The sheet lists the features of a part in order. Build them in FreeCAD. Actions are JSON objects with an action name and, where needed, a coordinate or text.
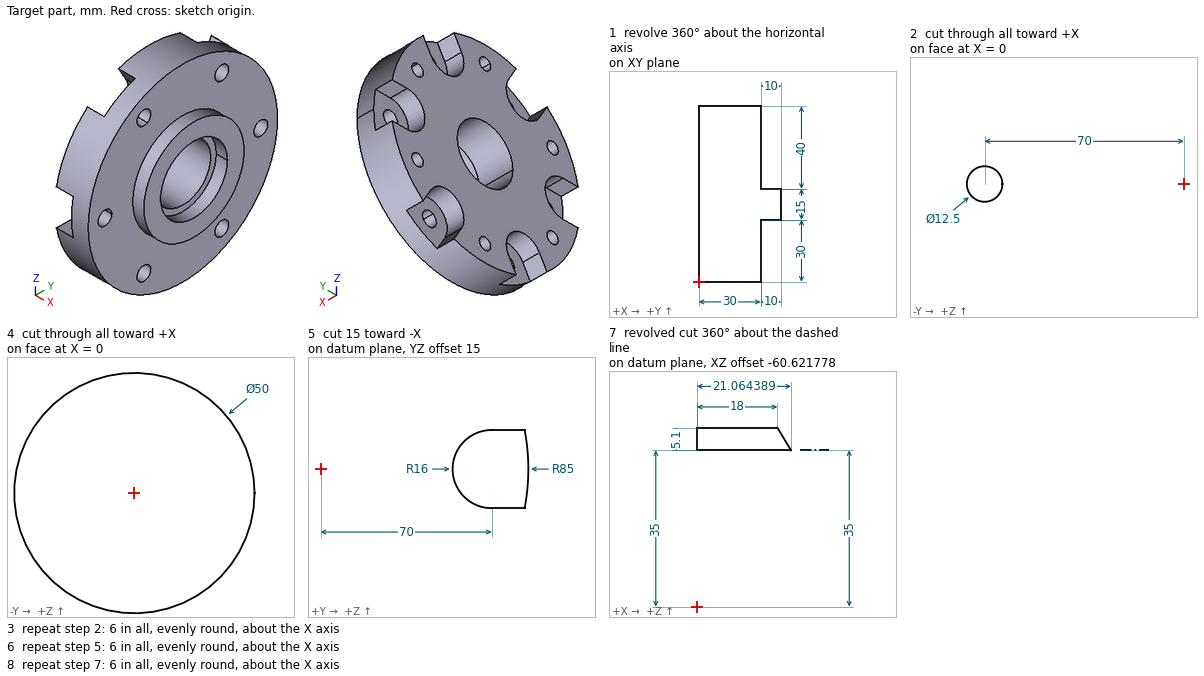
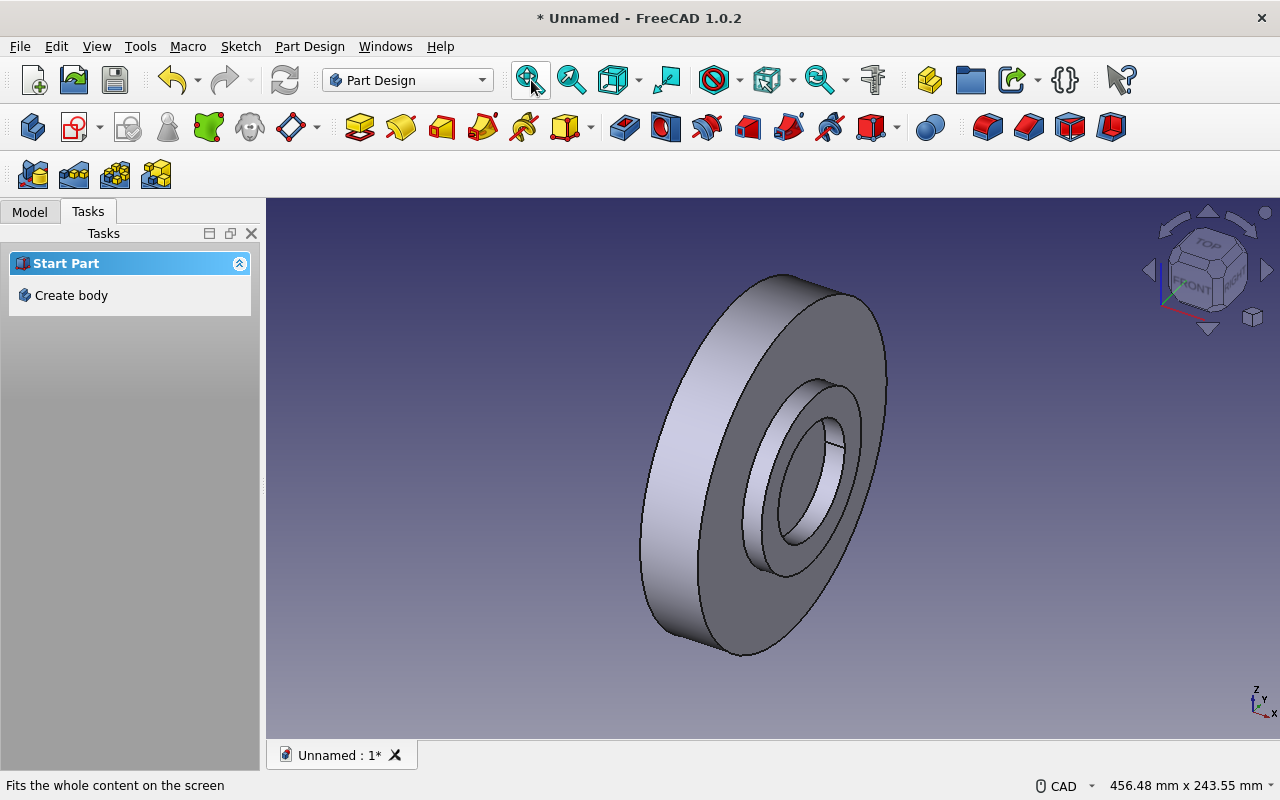
{"action": "key", "text": "6"}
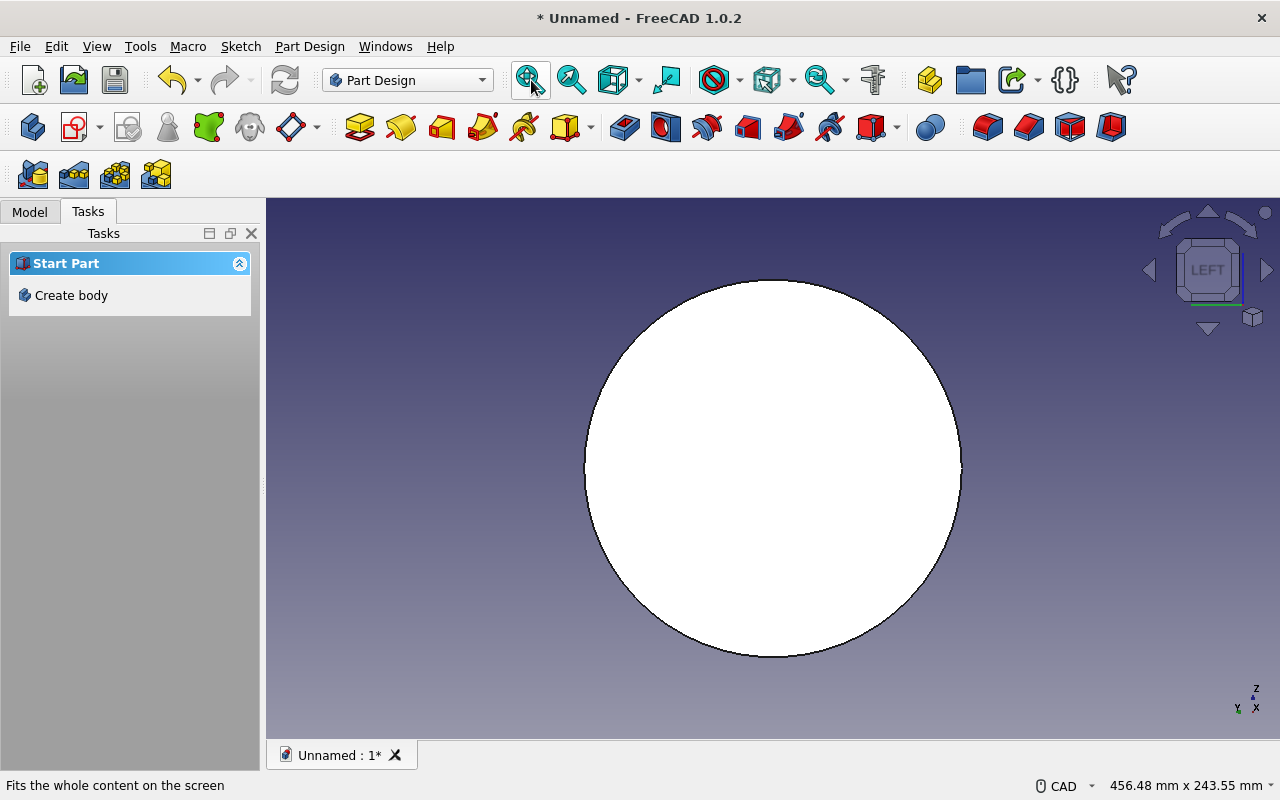
{"action": "left_click", "coordinate": [773, 467]}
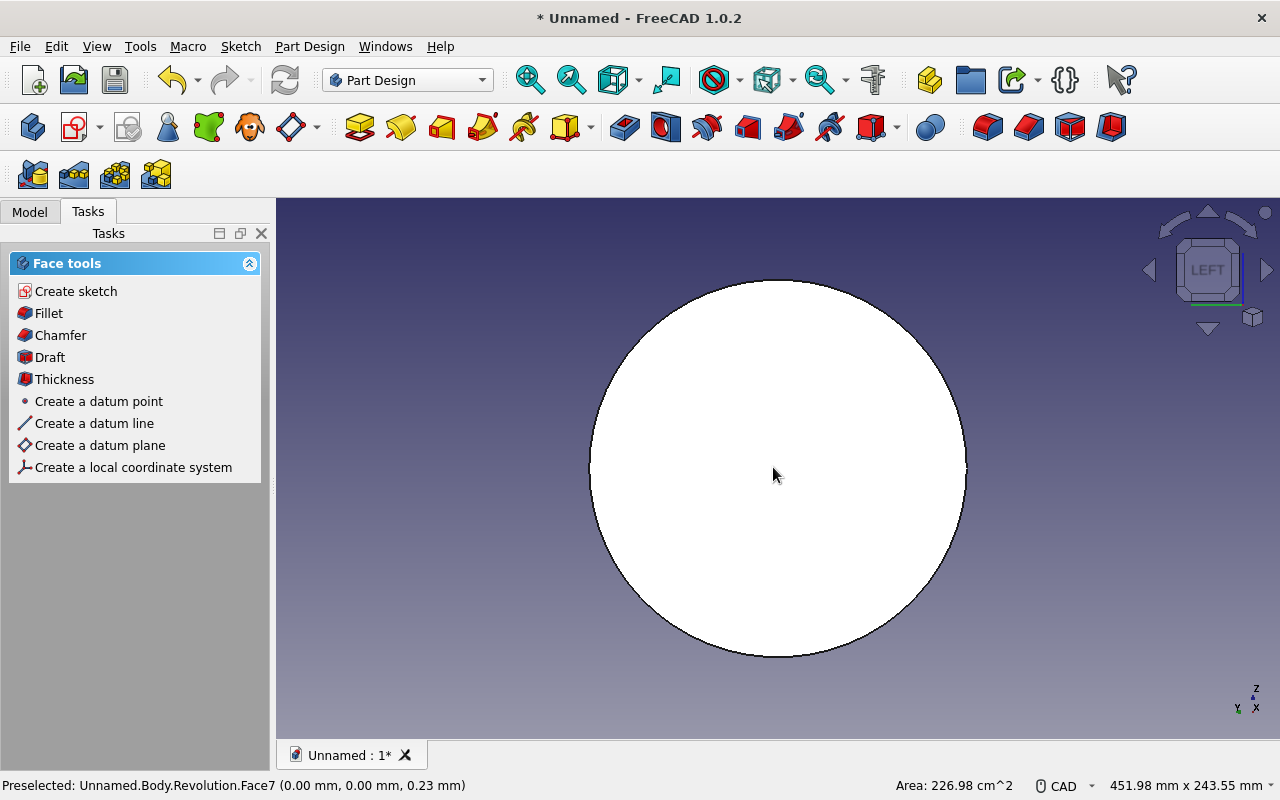
{"action": "left_click", "coordinate": [74, 128]}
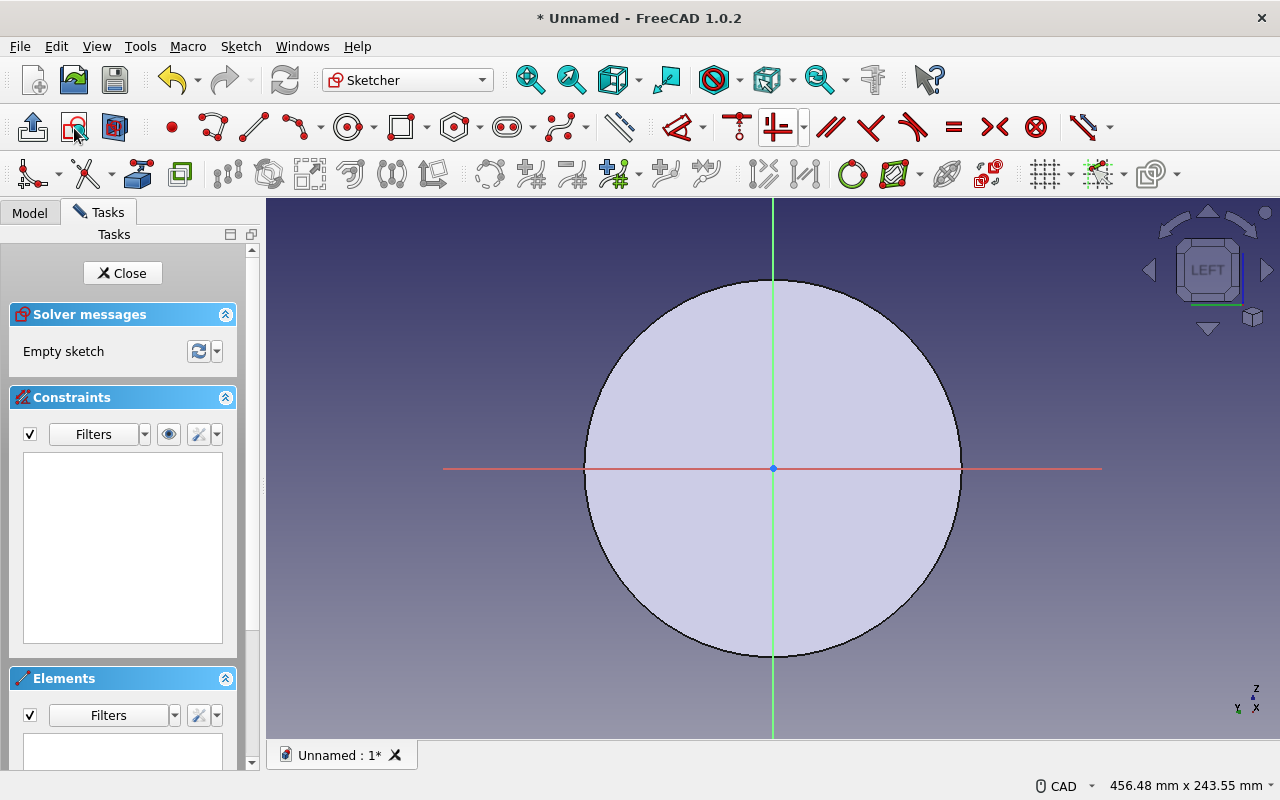
{"action": "scroll", "coordinate": [611, 468], "scroll_direction": "up", "scroll_amount": 13}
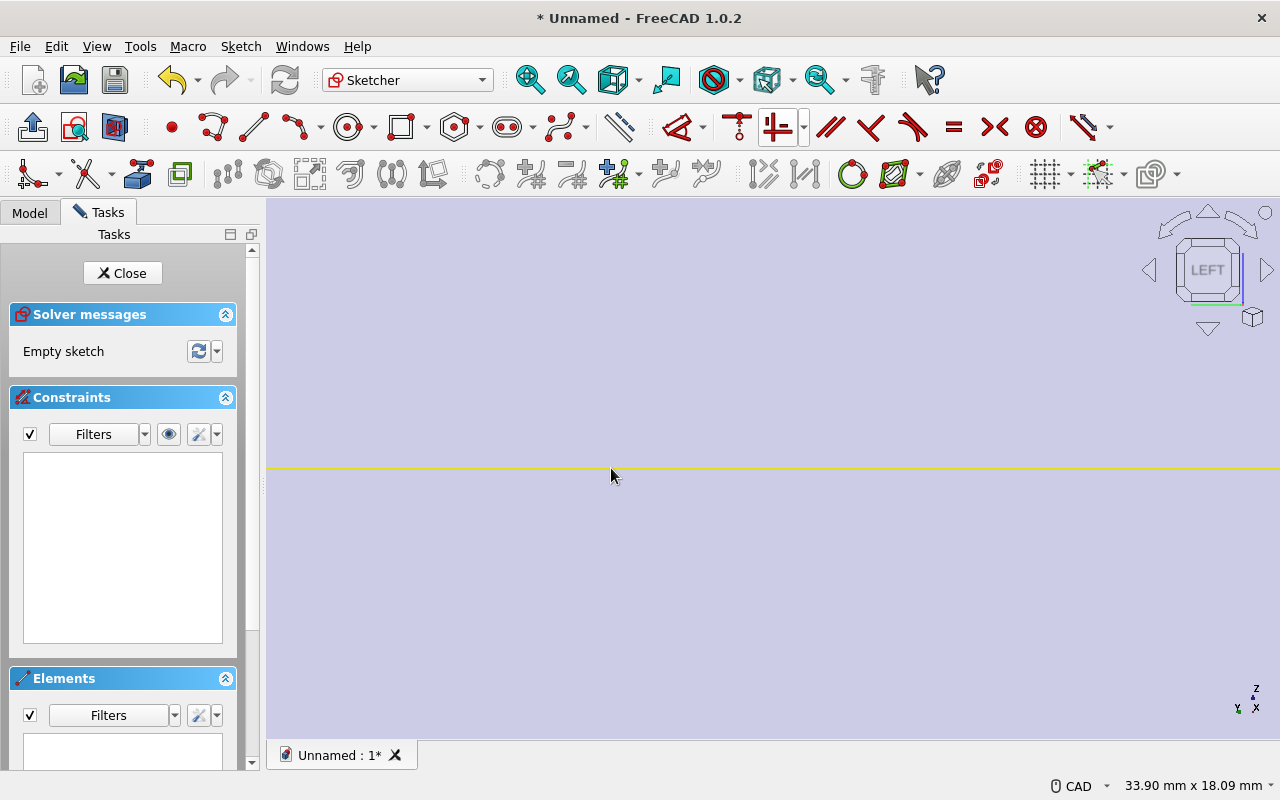
{"action": "left_click", "coordinate": [348, 128]}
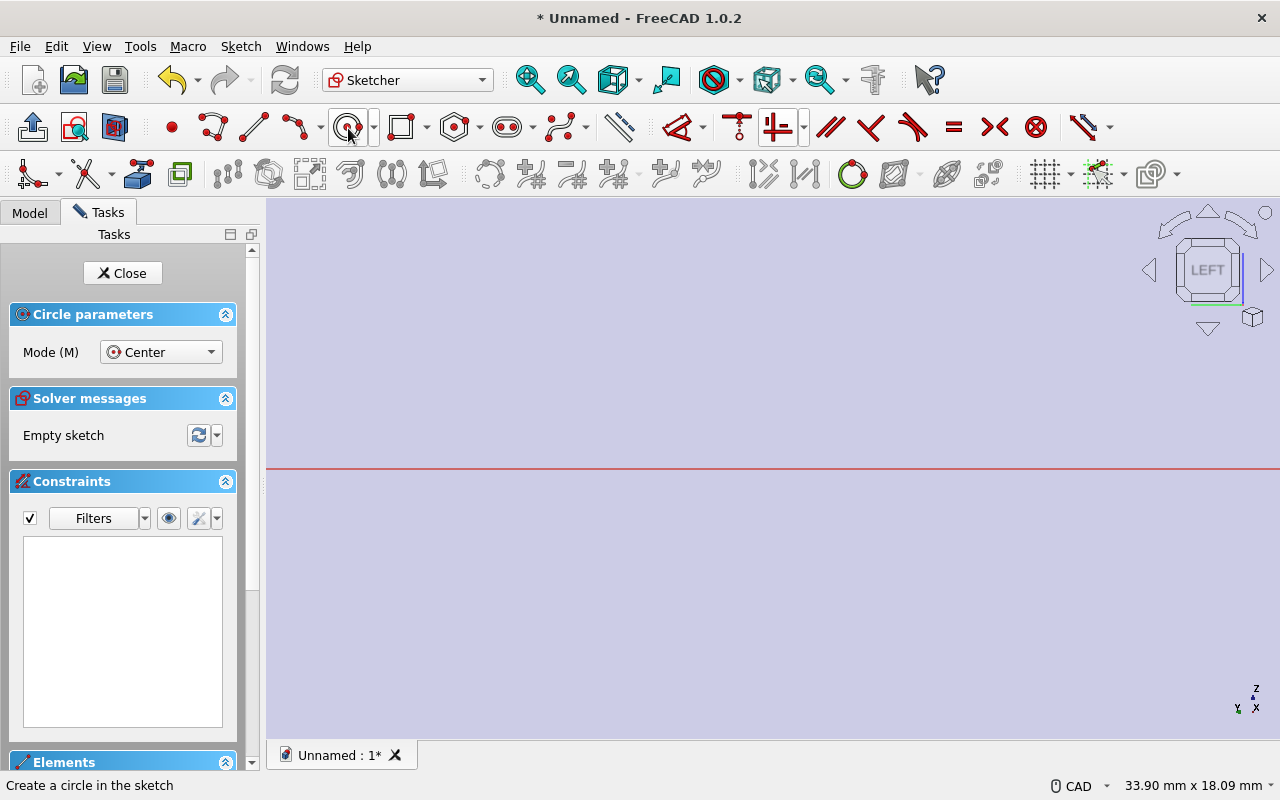
{"action": "left_click", "coordinate": [694, 468]}
{"action": "left_click", "coordinate": [827, 336]}
{"action": "key", "text": "Escape"}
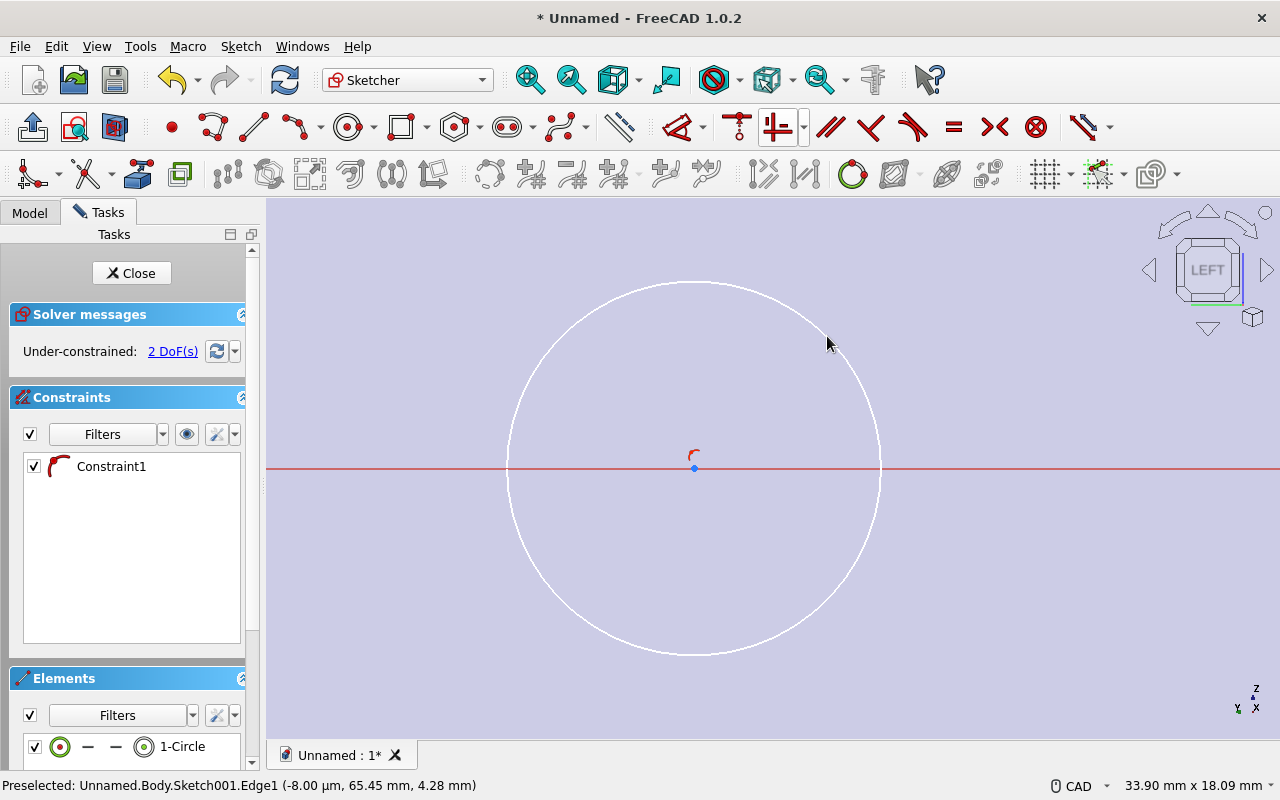
{"action": "left_click", "coordinate": [676, 128]}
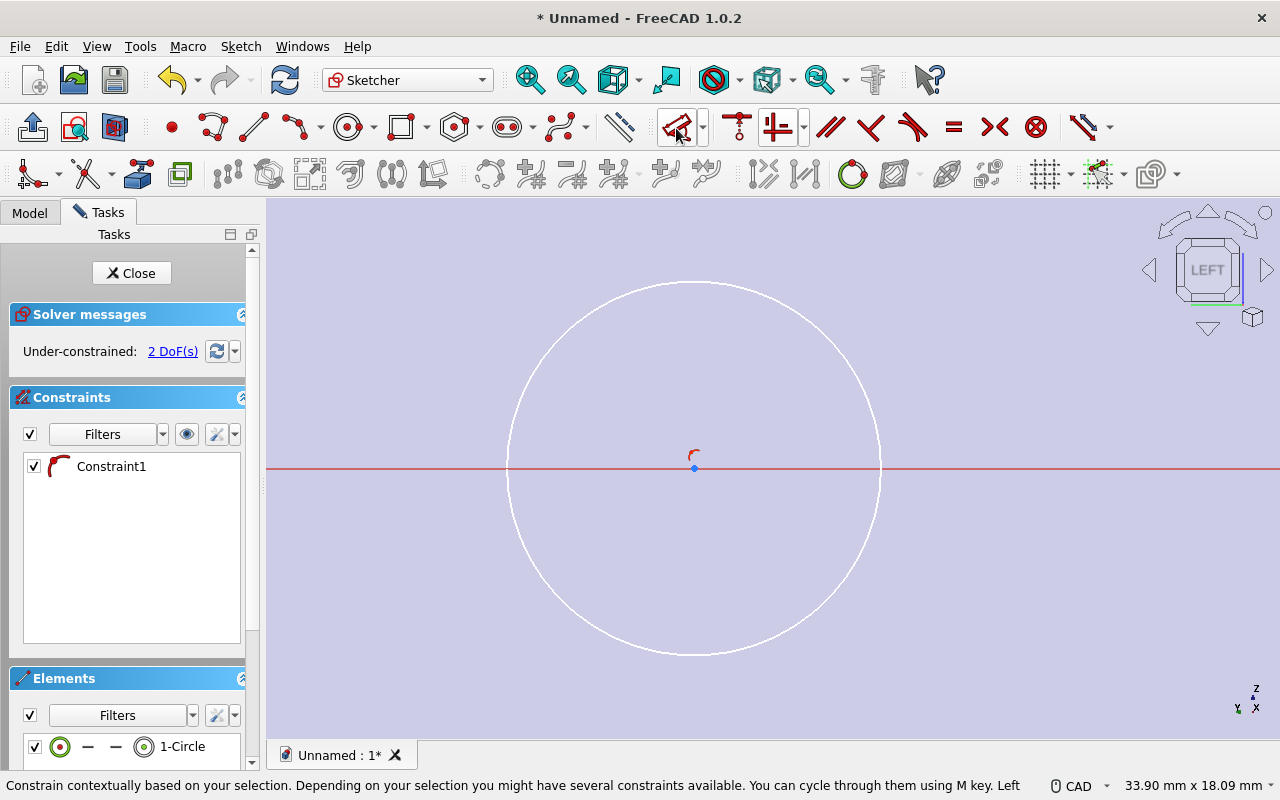
{"action": "left_click", "coordinate": [826, 336]}
{"action": "left_click", "coordinate": [849, 313]}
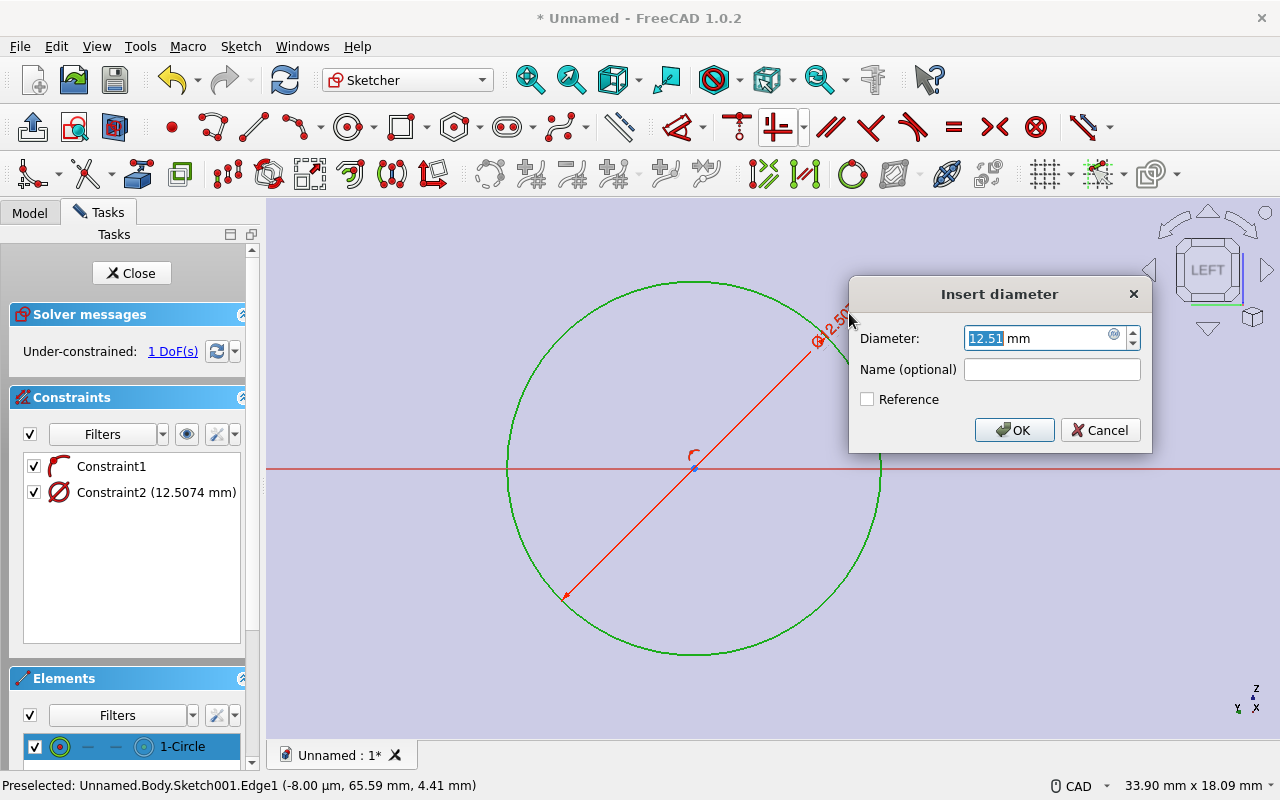
{"action": "type", "text": "12.5"}
{"action": "key", "text": "Return"}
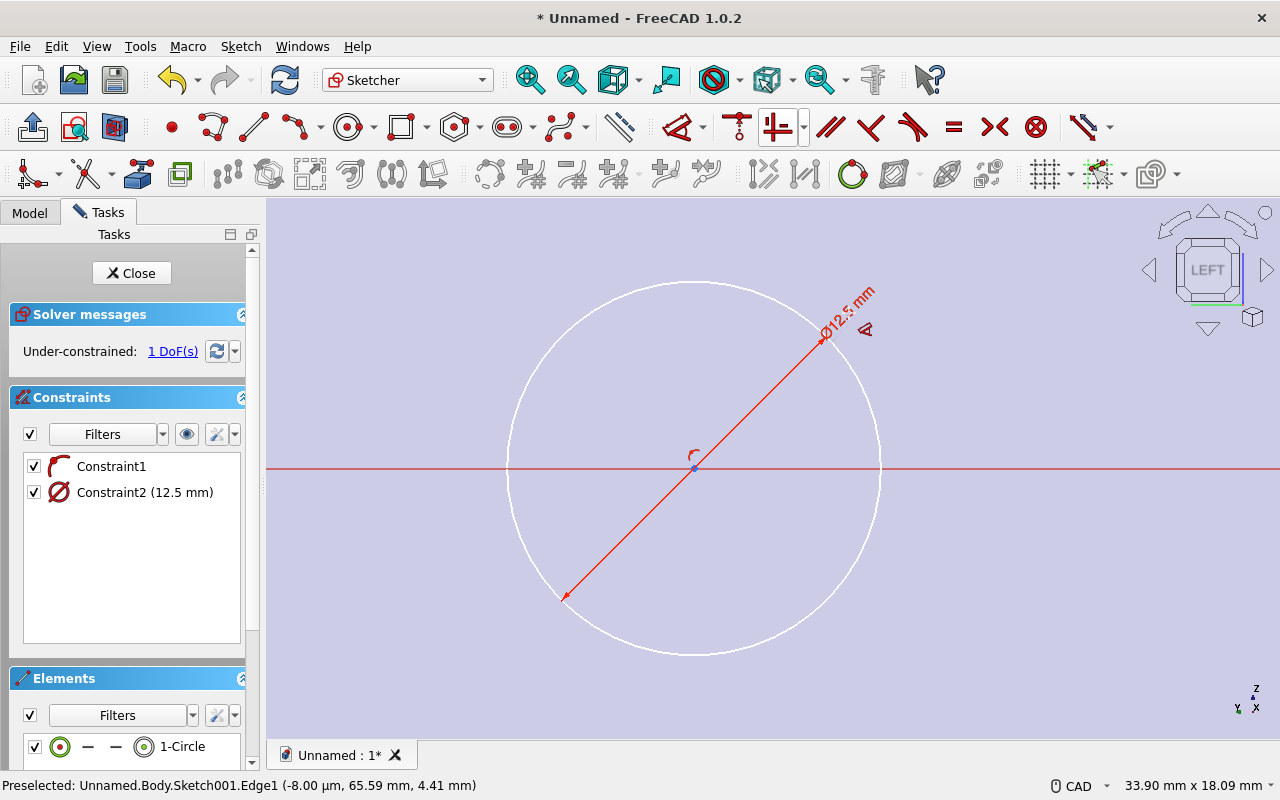
{"action": "left_click", "coordinate": [694, 468]}
{"action": "left_click", "coordinate": [905, 502]}